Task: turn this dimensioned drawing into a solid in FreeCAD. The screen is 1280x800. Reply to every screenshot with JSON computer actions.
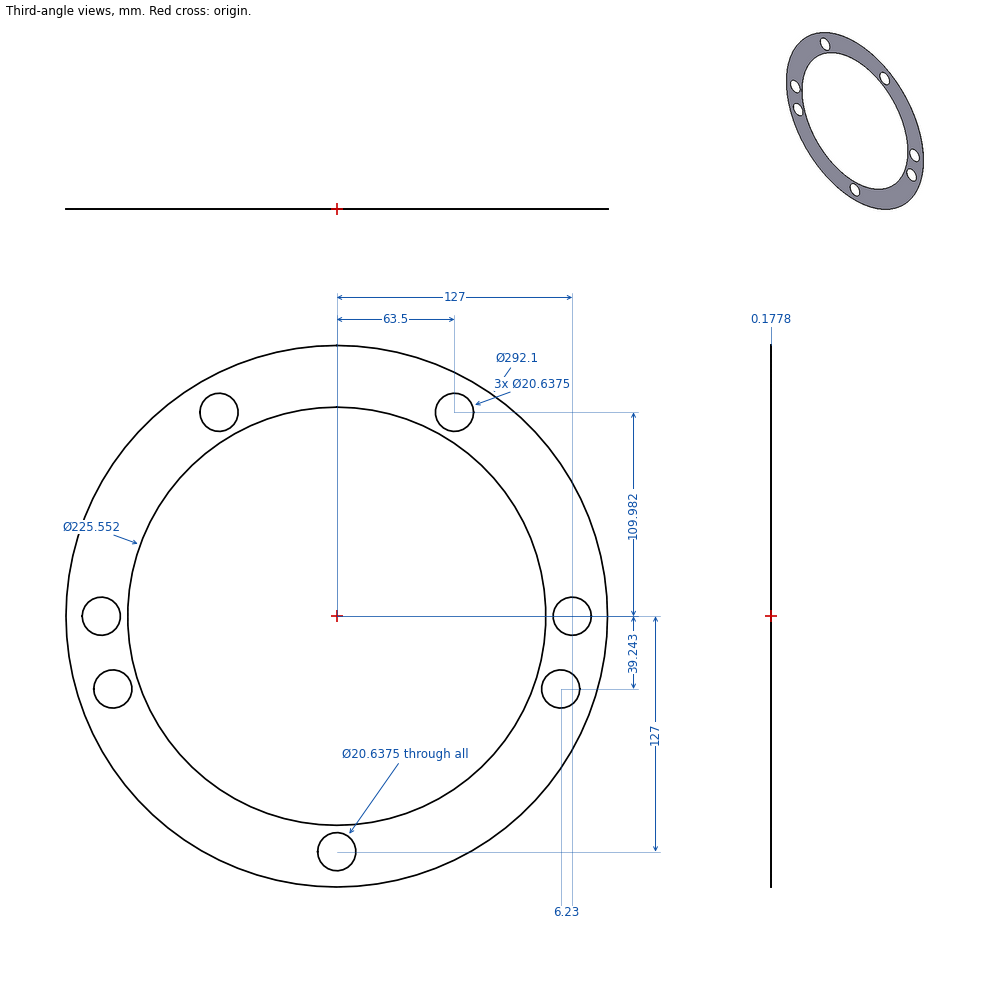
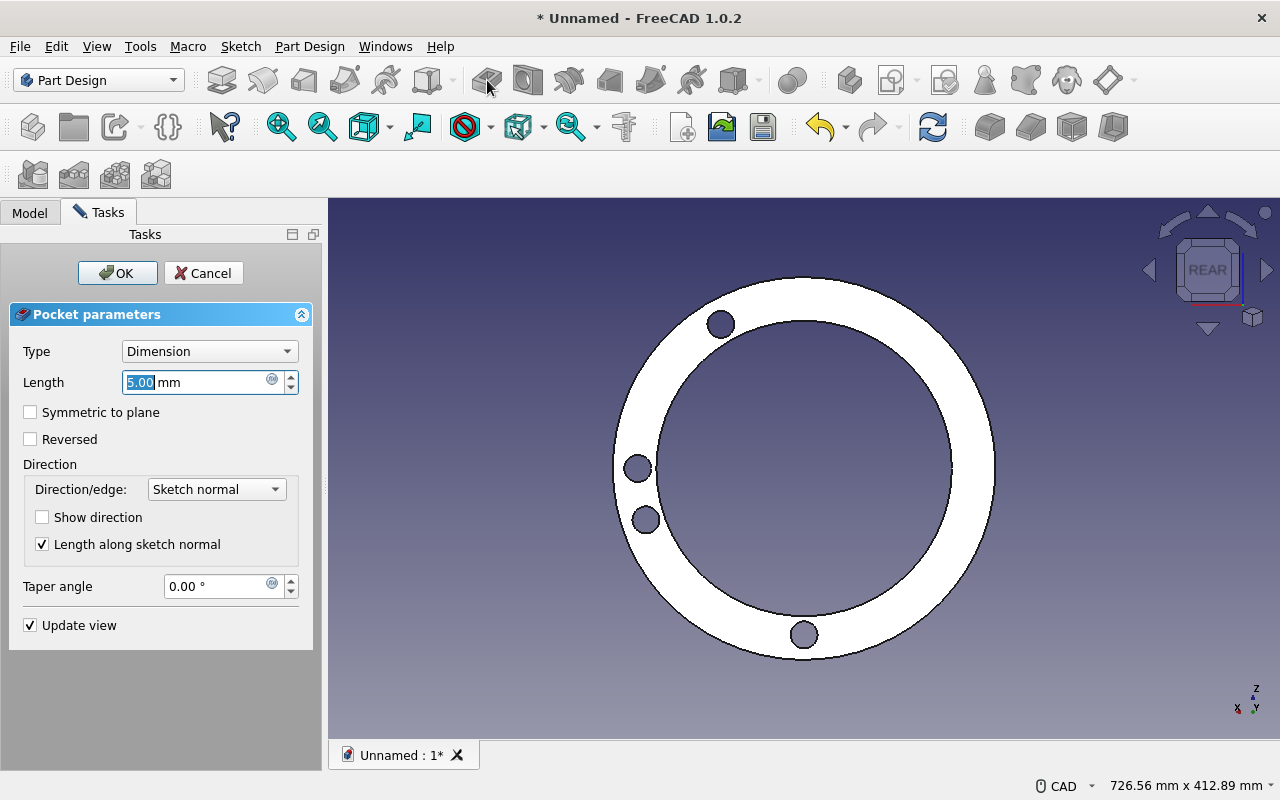
{"action": "left_click", "coordinate": [210, 352]}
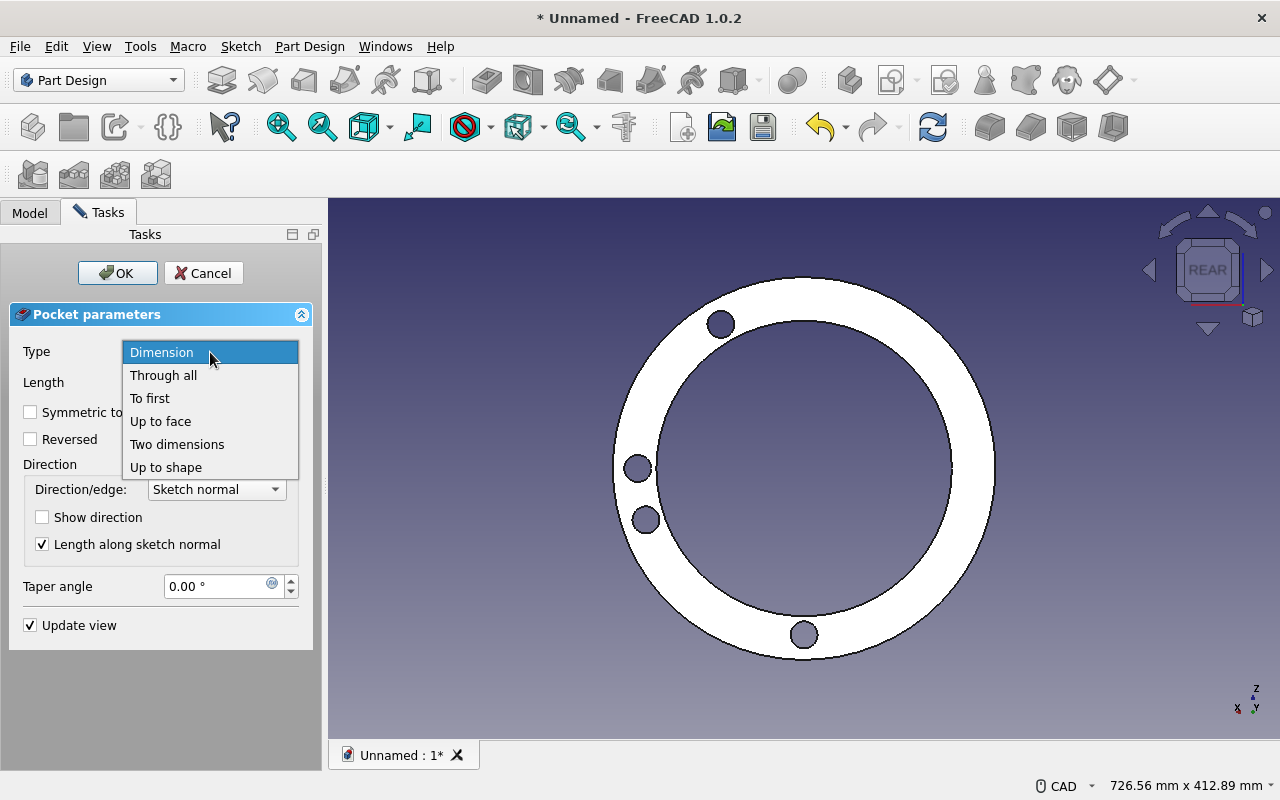
{"action": "left_click", "coordinate": [208, 376]}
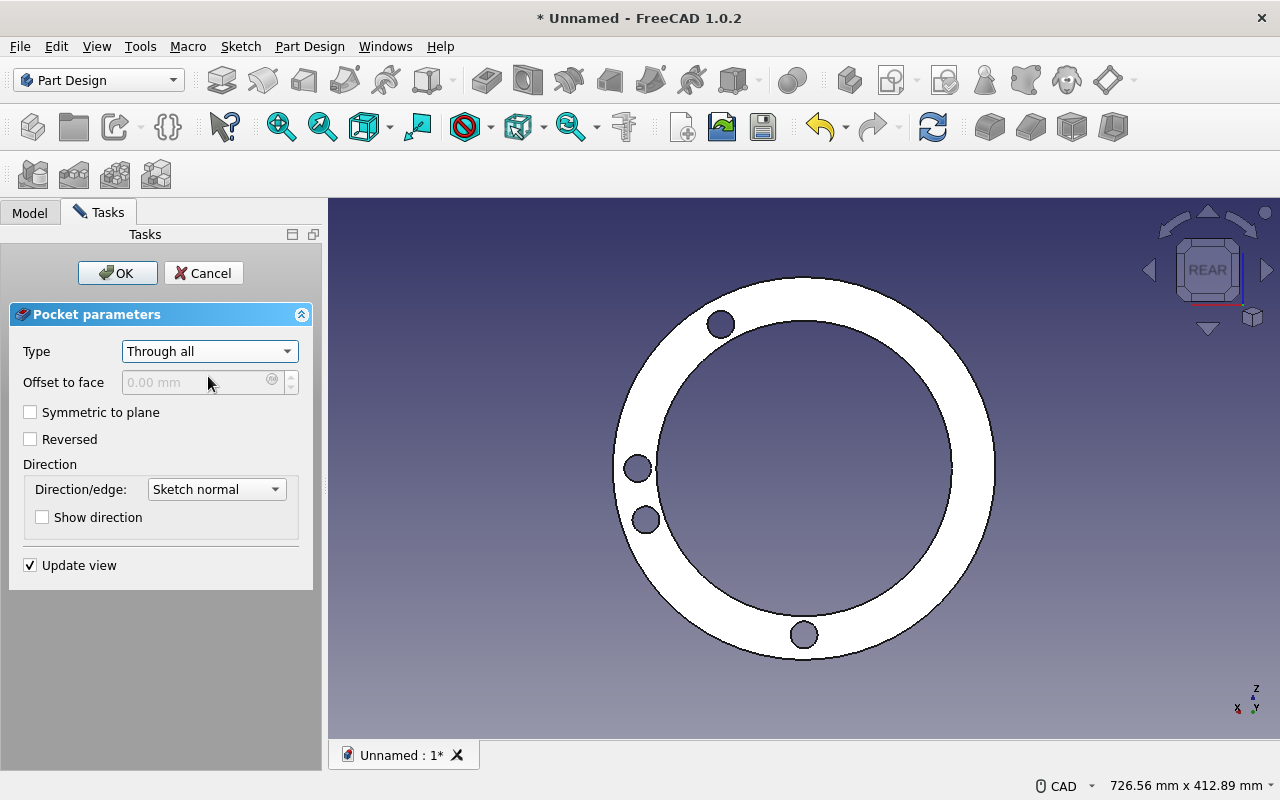
{"action": "left_click", "coordinate": [118, 273]}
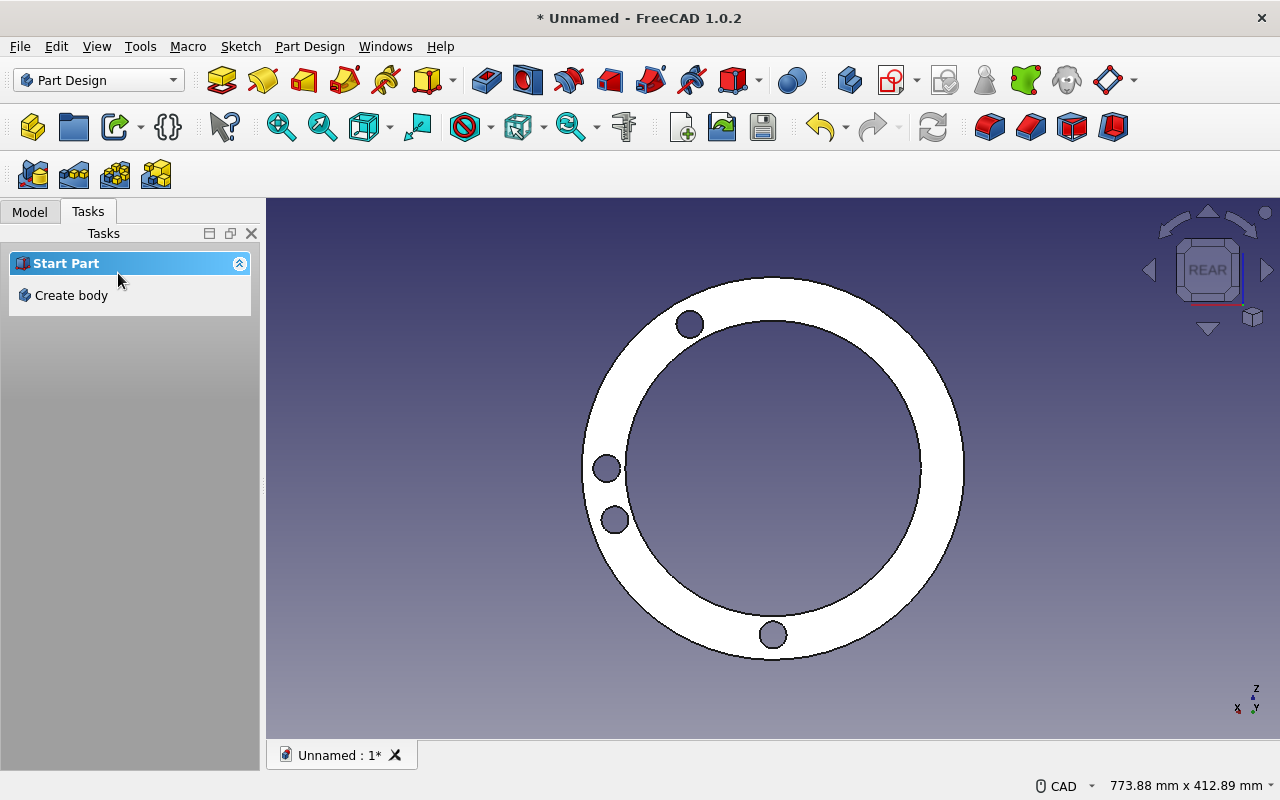
{"action": "left_click", "coordinate": [30, 212]}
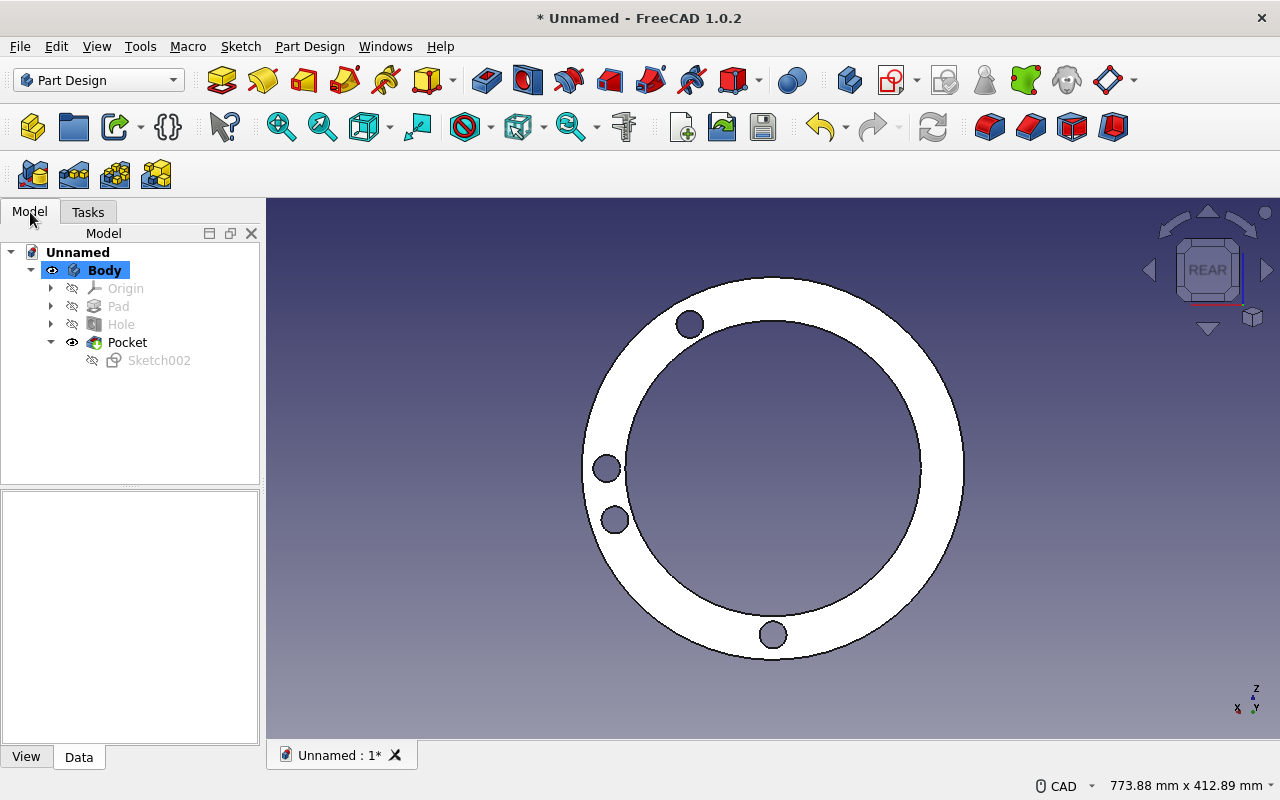
{"action": "left_click", "coordinate": [117, 342]}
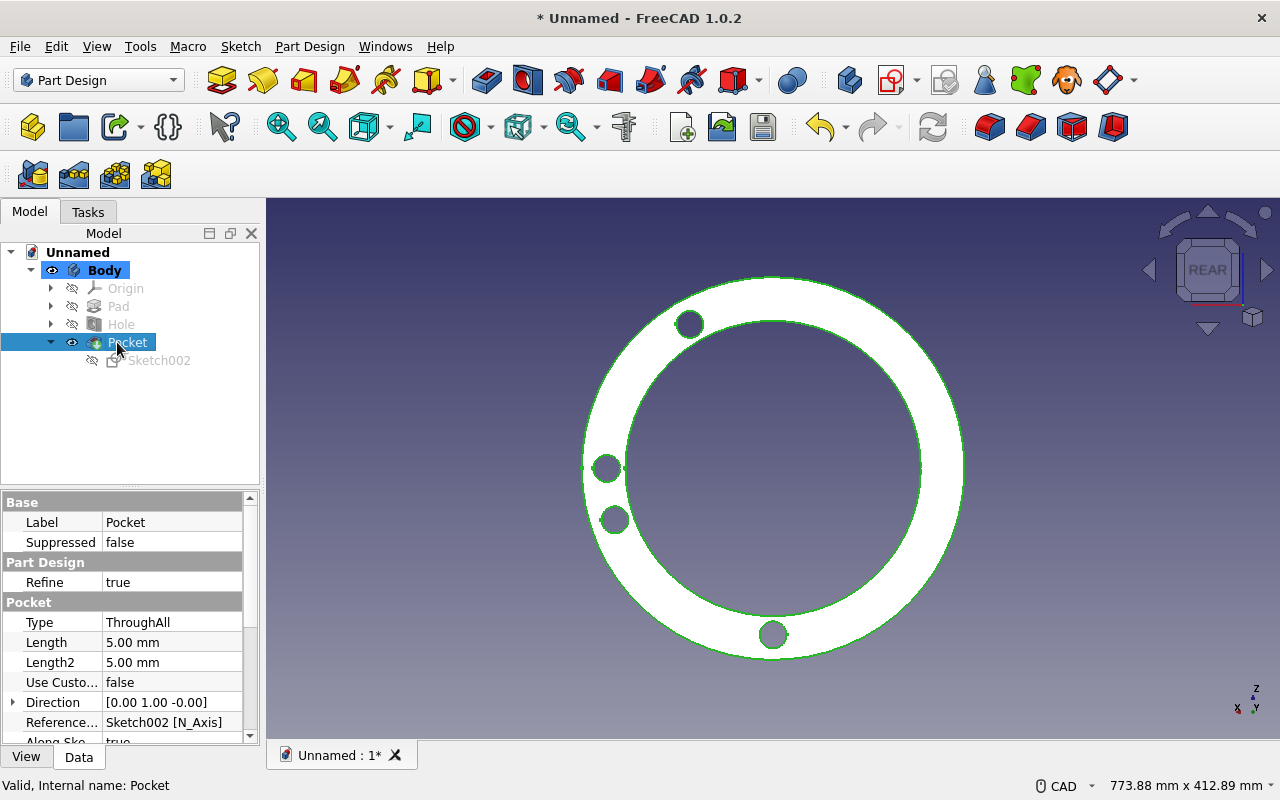
{"action": "left_click", "coordinate": [33, 174]}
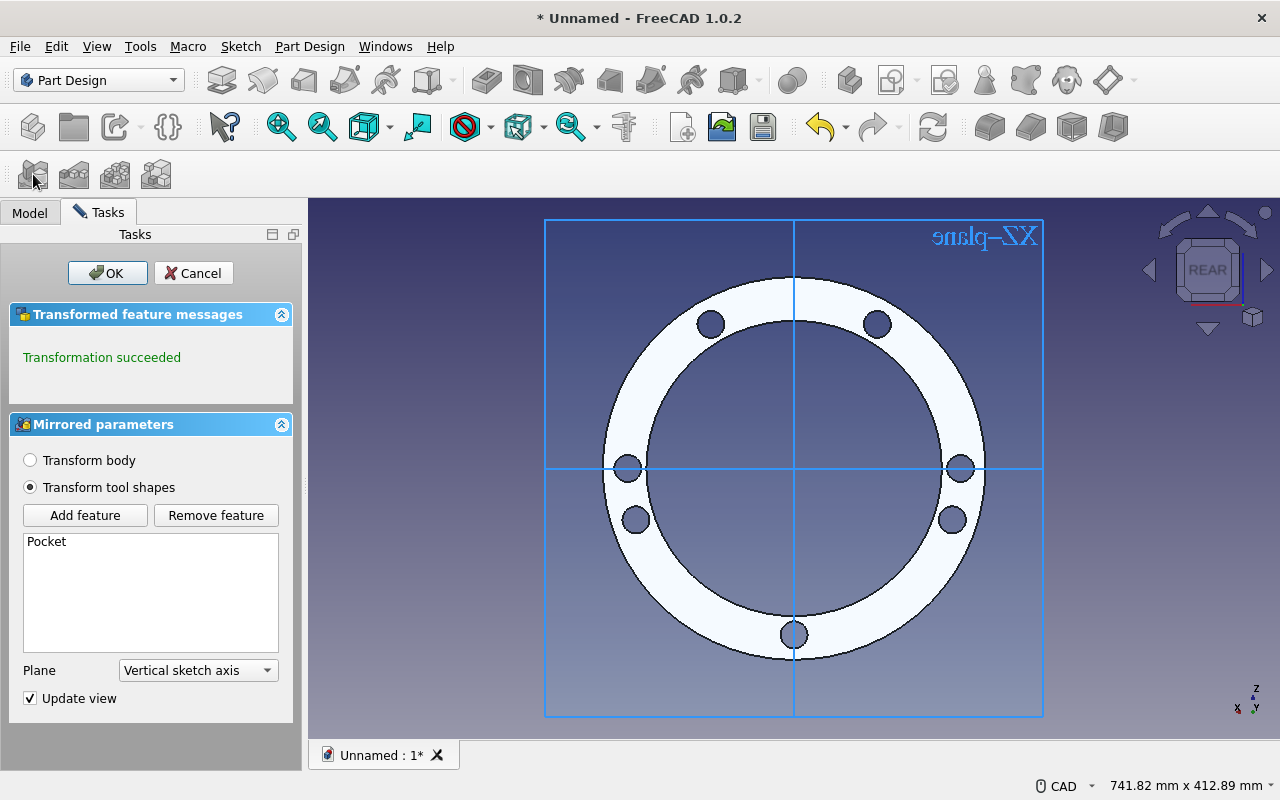
{"action": "left_click", "coordinate": [199, 670]}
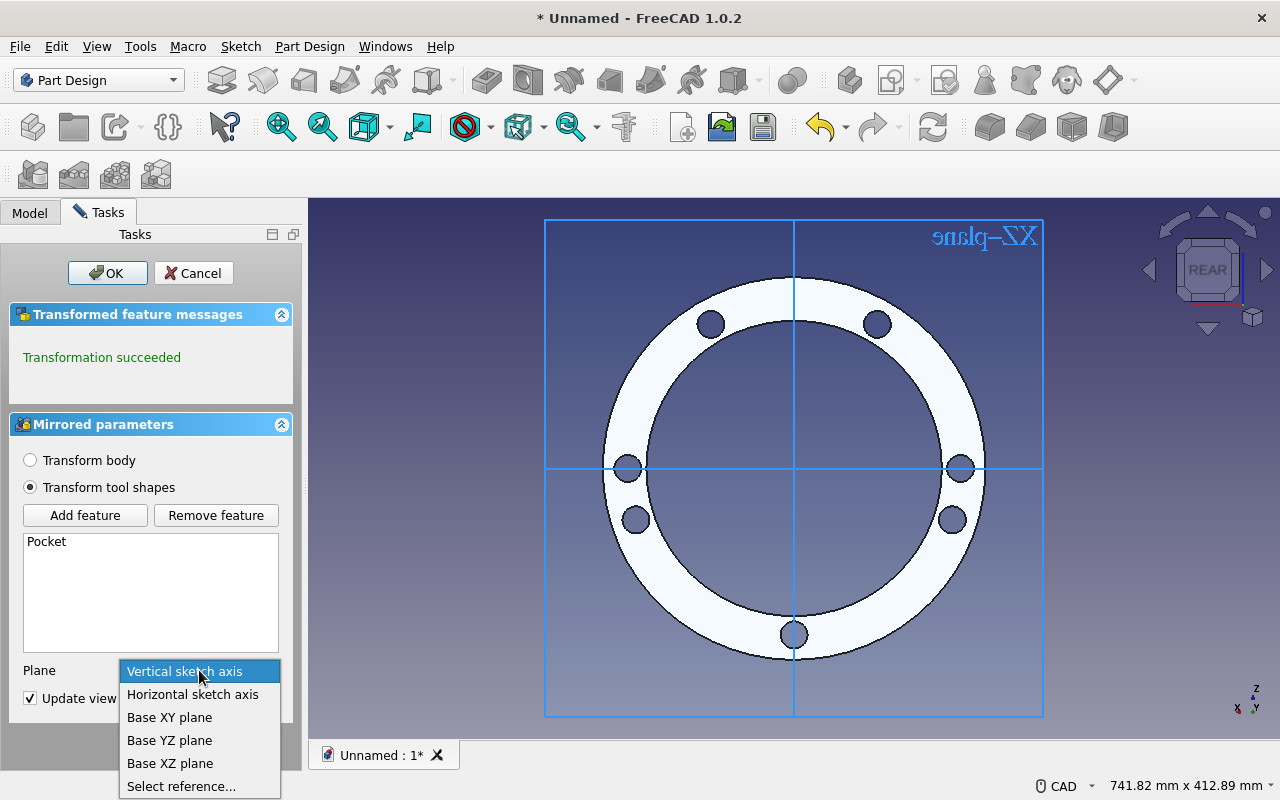
{"action": "left_click", "coordinate": [198, 740]}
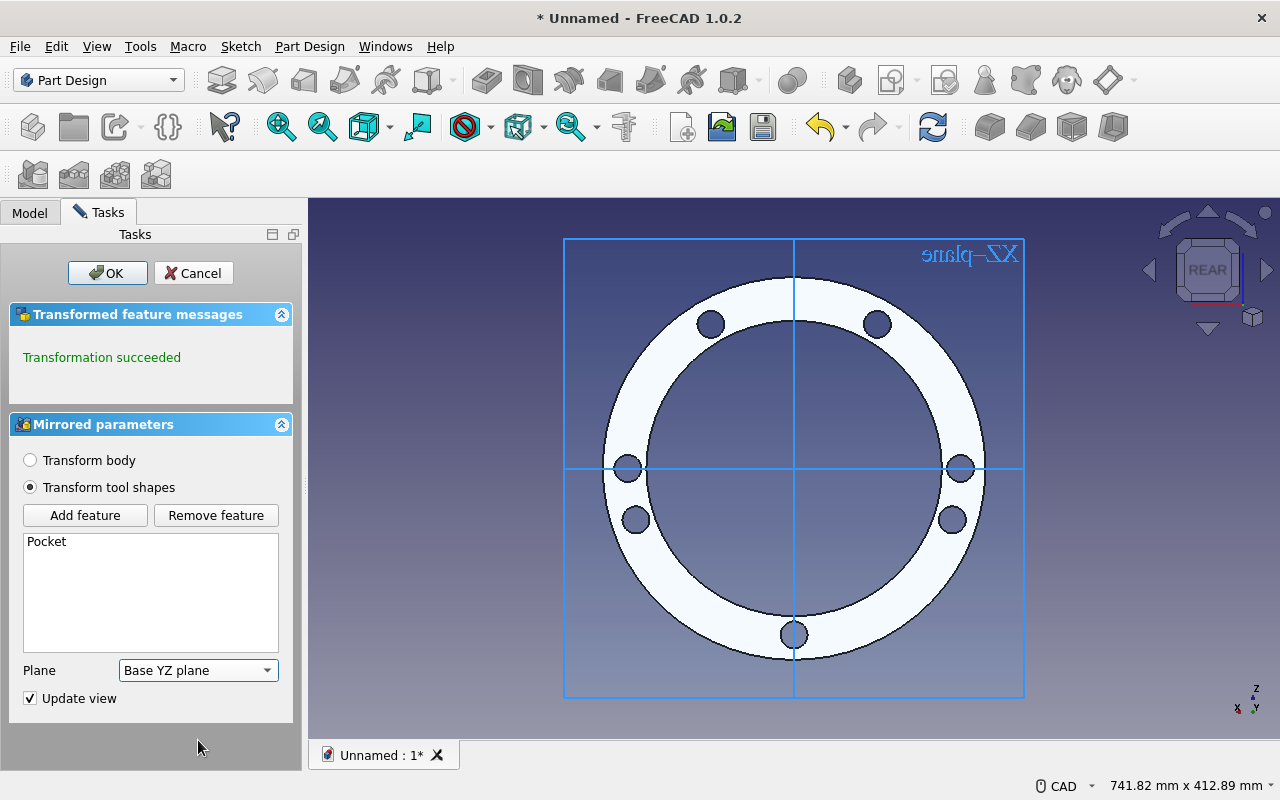
{"action": "left_click", "coordinate": [108, 273]}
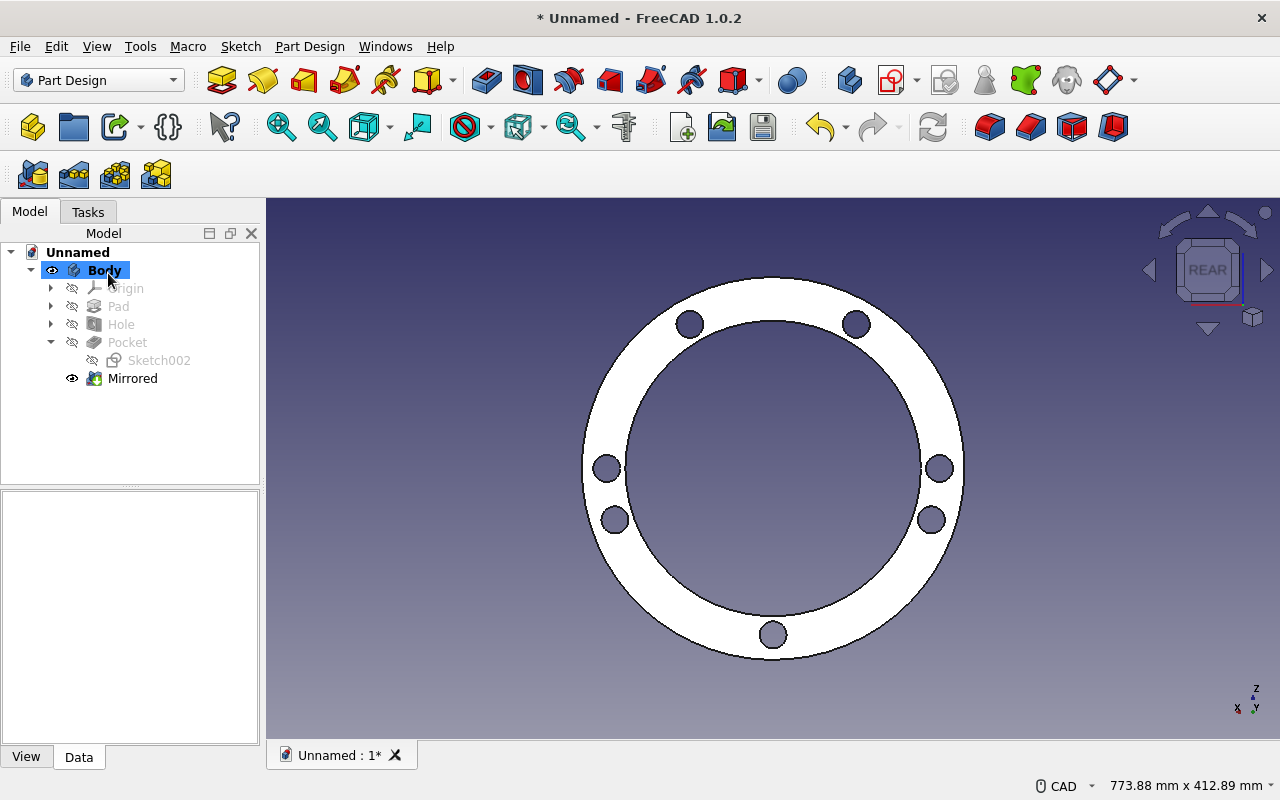
{"action": "key", "text": "0"}